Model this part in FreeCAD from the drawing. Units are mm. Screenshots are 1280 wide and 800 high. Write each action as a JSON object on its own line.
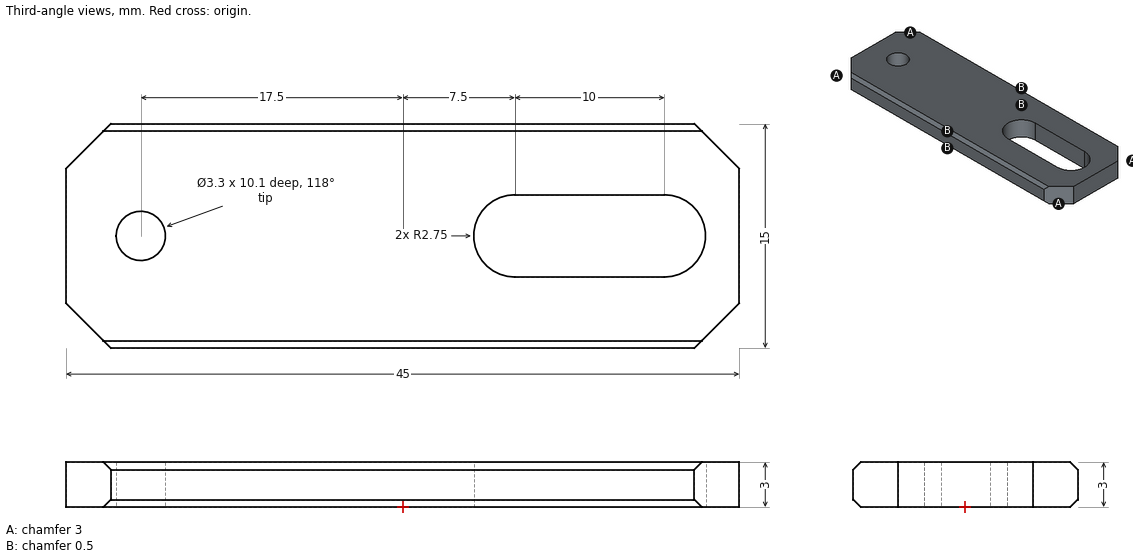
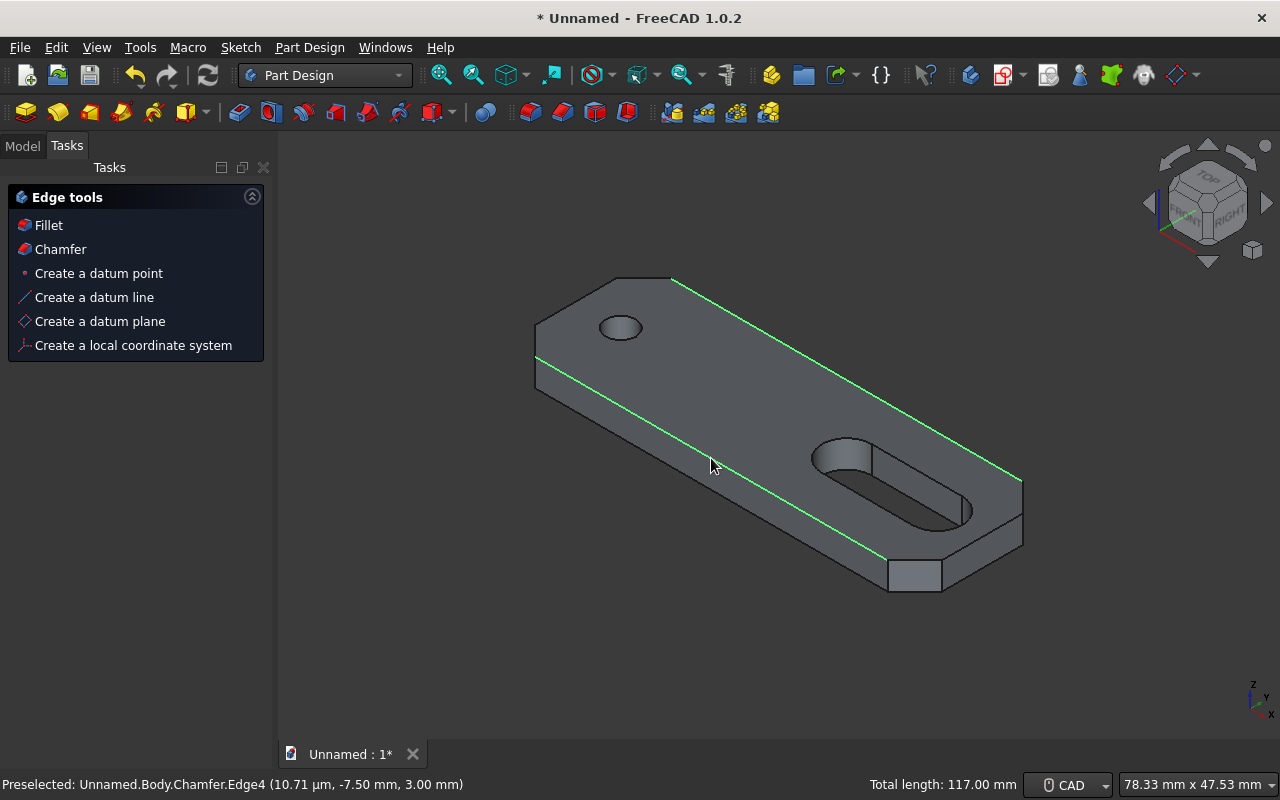
{"action": "key", "text": "2"}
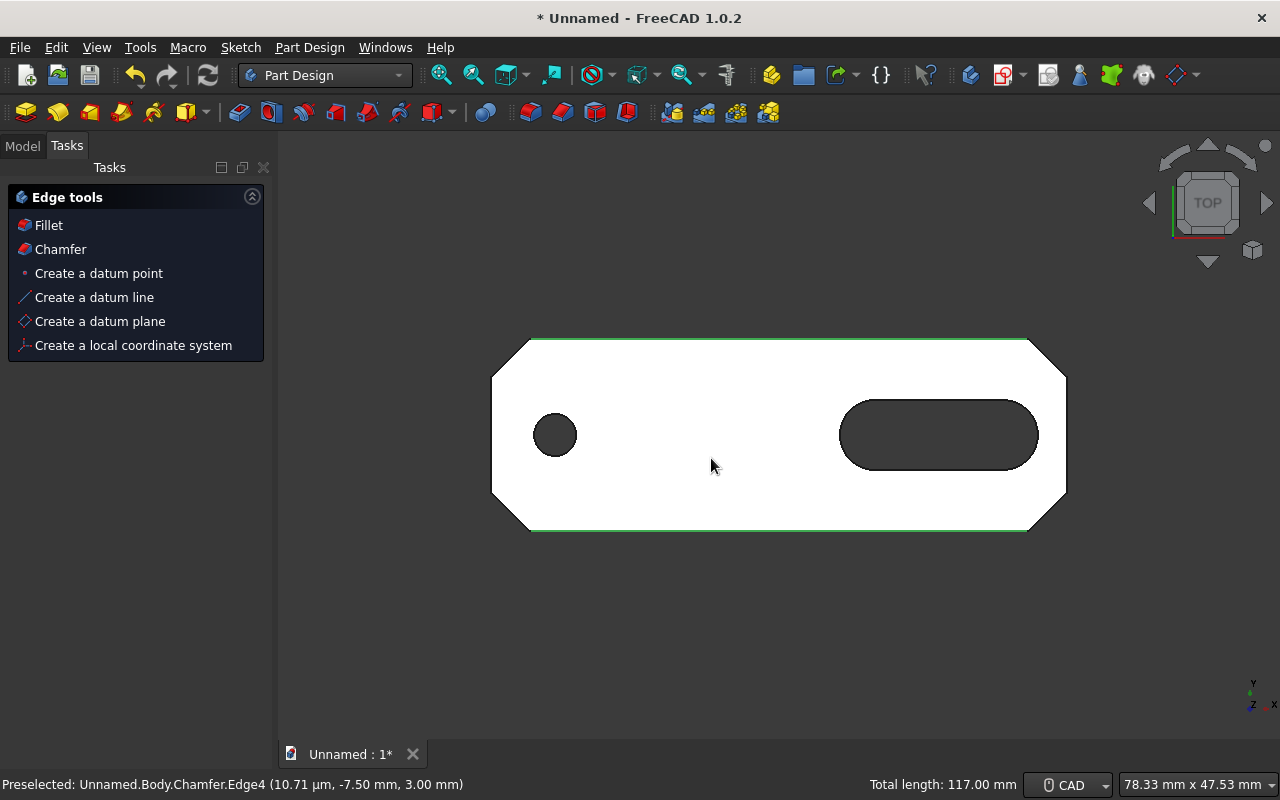
{"action": "key", "text": "1"}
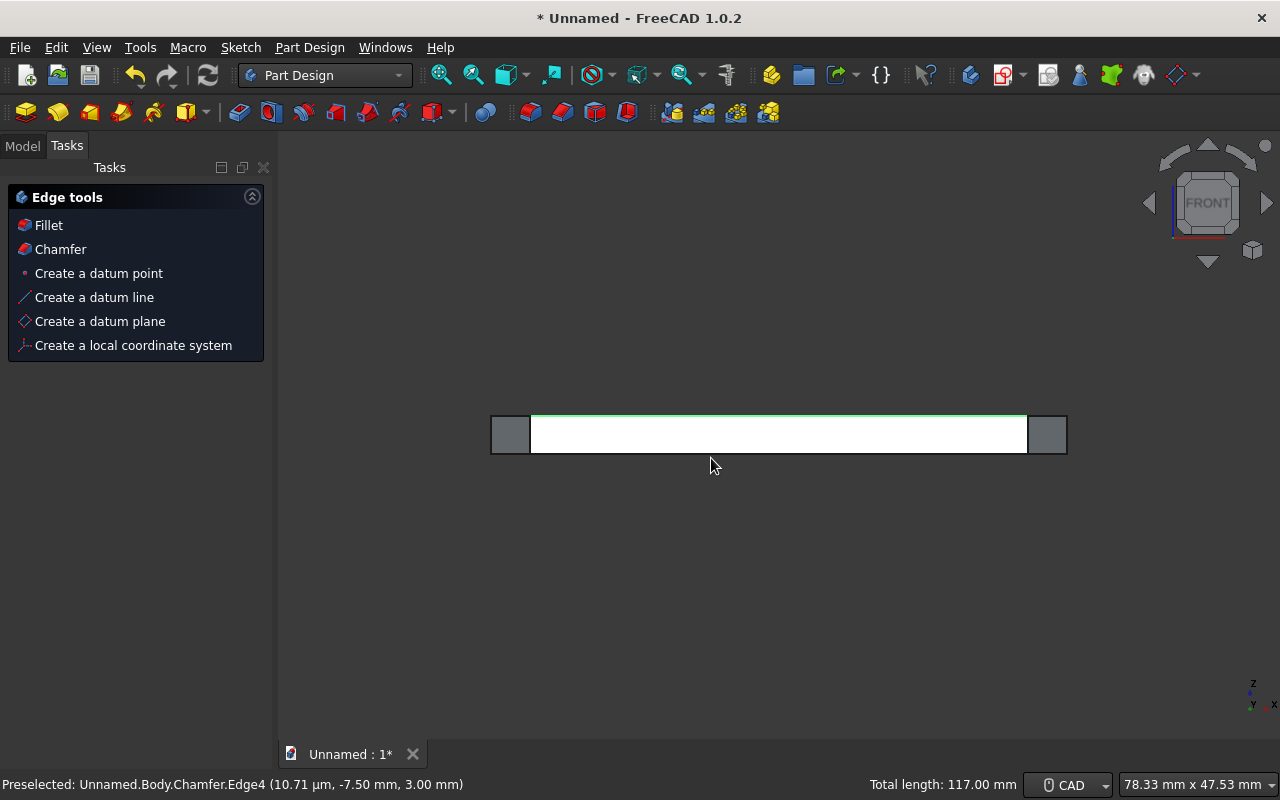
{"action": "left_click", "coordinate": [779, 453], "text": "ctrl"}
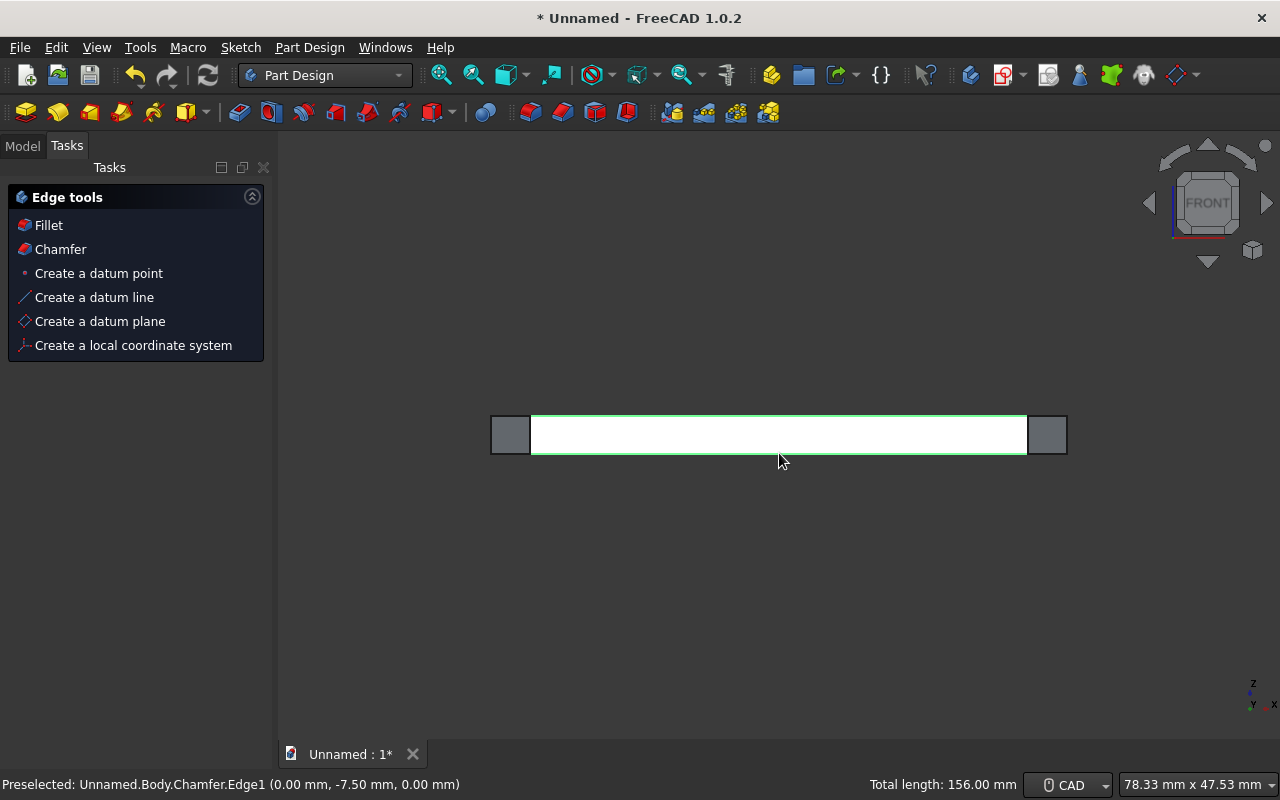
{"action": "left_click", "coordinate": [564, 112]}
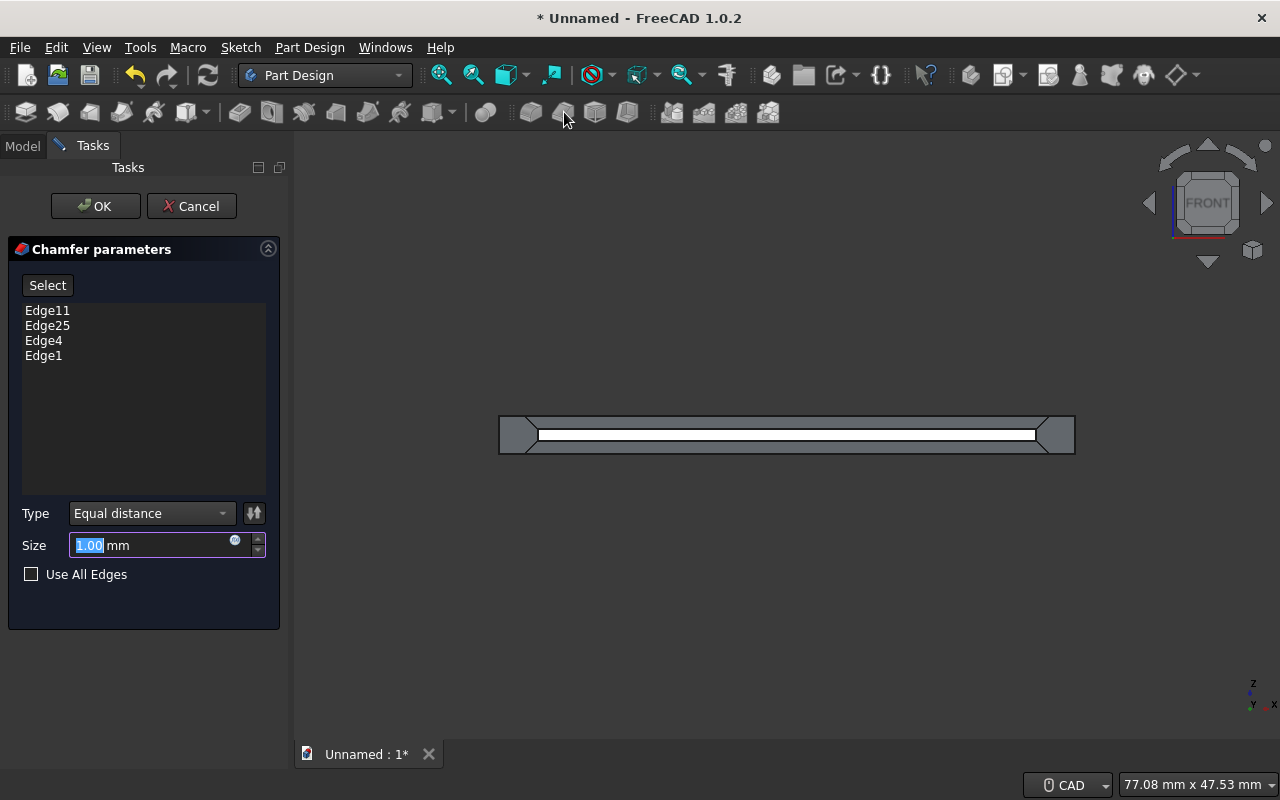
{"action": "type", "text": "0.5"}
{"action": "key", "text": "Tab"}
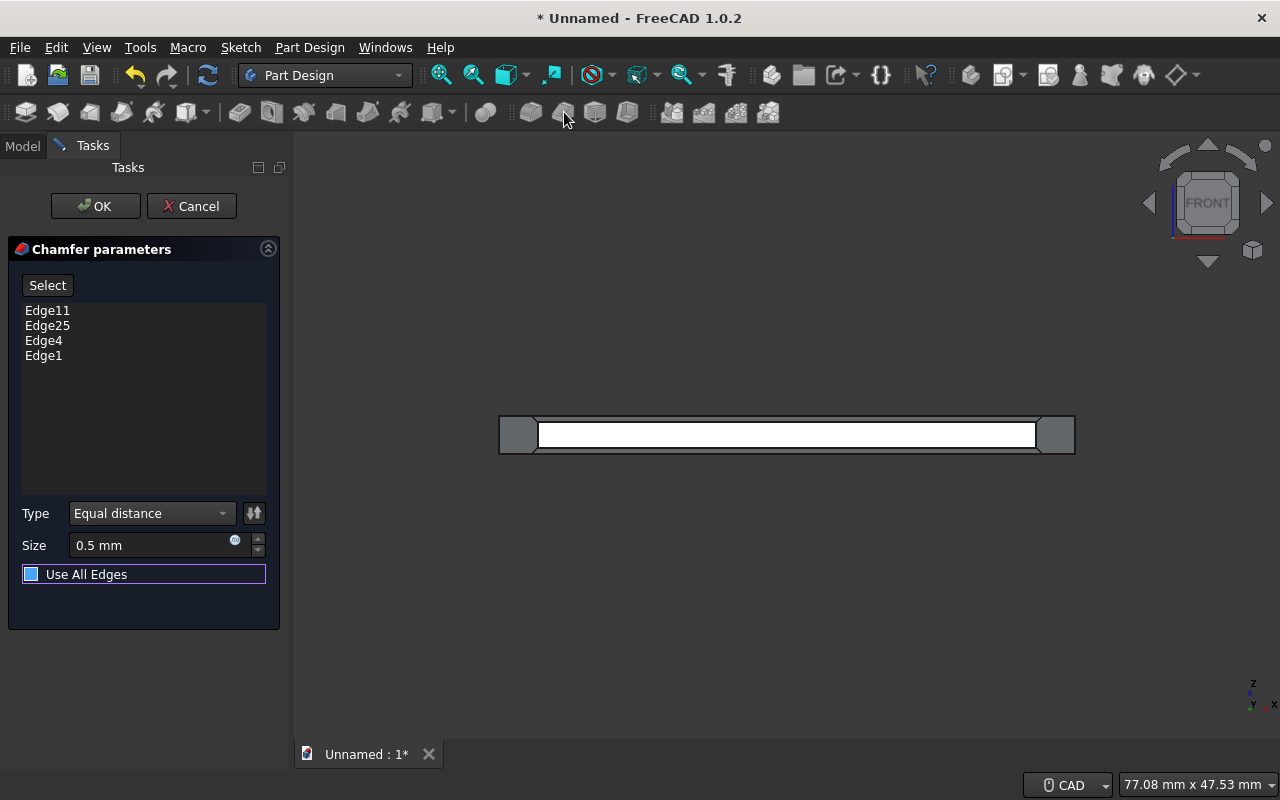
{"action": "left_click", "coordinate": [96, 206]}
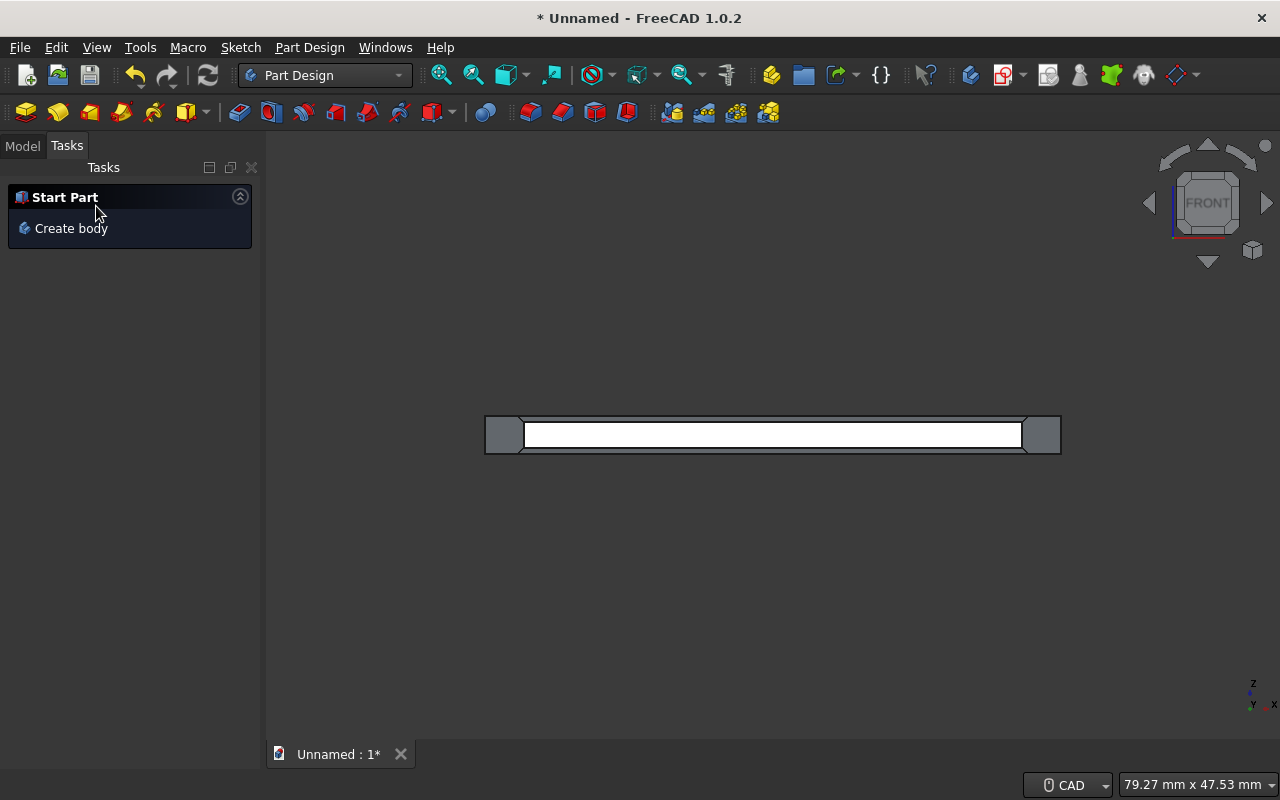
{"action": "key", "text": "0"}